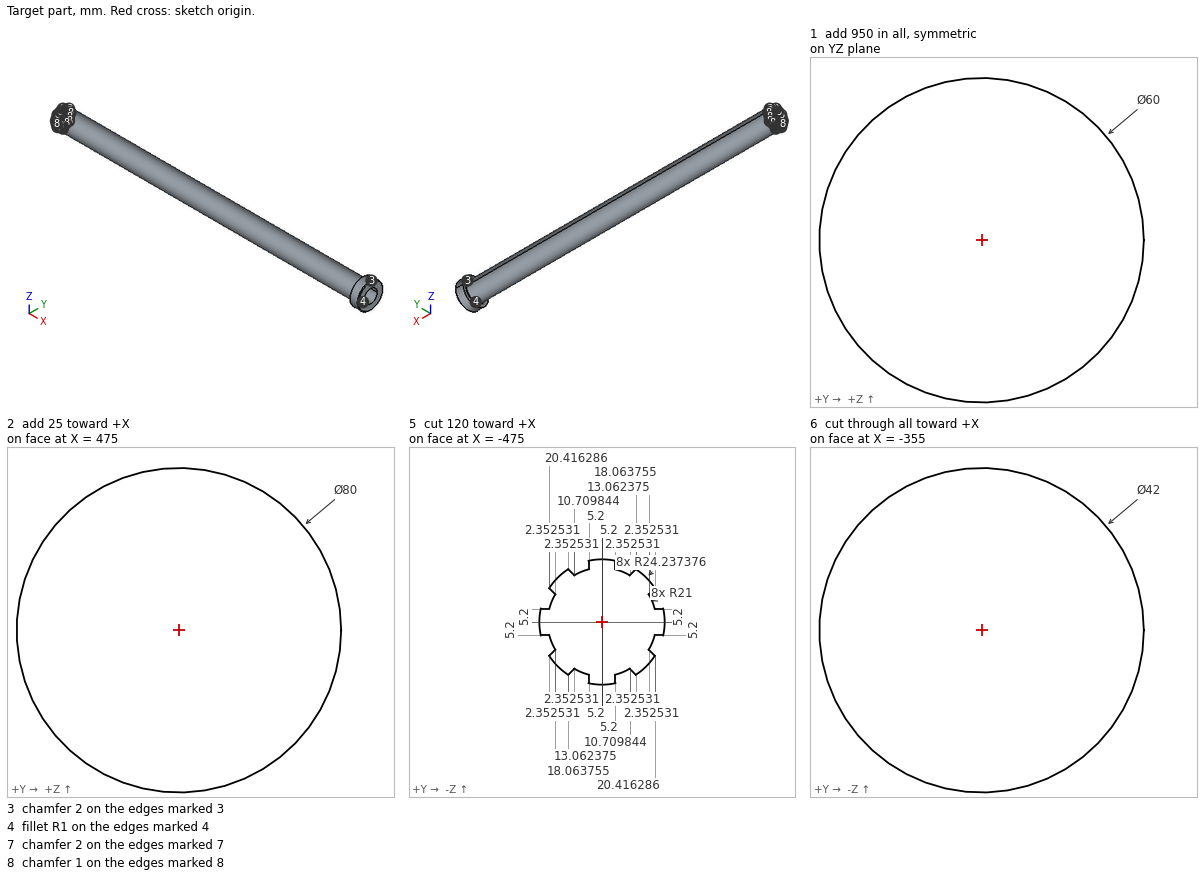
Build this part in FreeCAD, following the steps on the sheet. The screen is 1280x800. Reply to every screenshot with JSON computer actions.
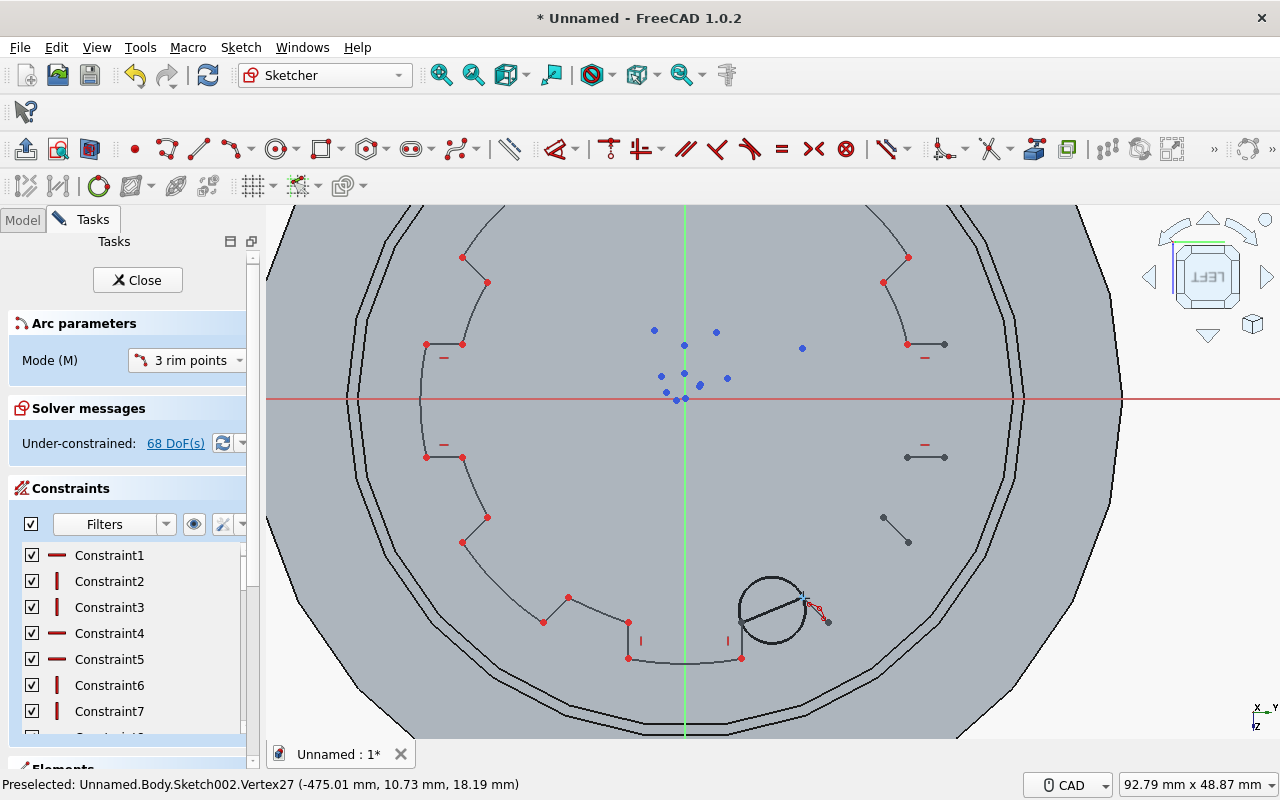
{"action": "scroll", "coordinate": [773, 611], "scroll_direction": "up", "scroll_amount": 10}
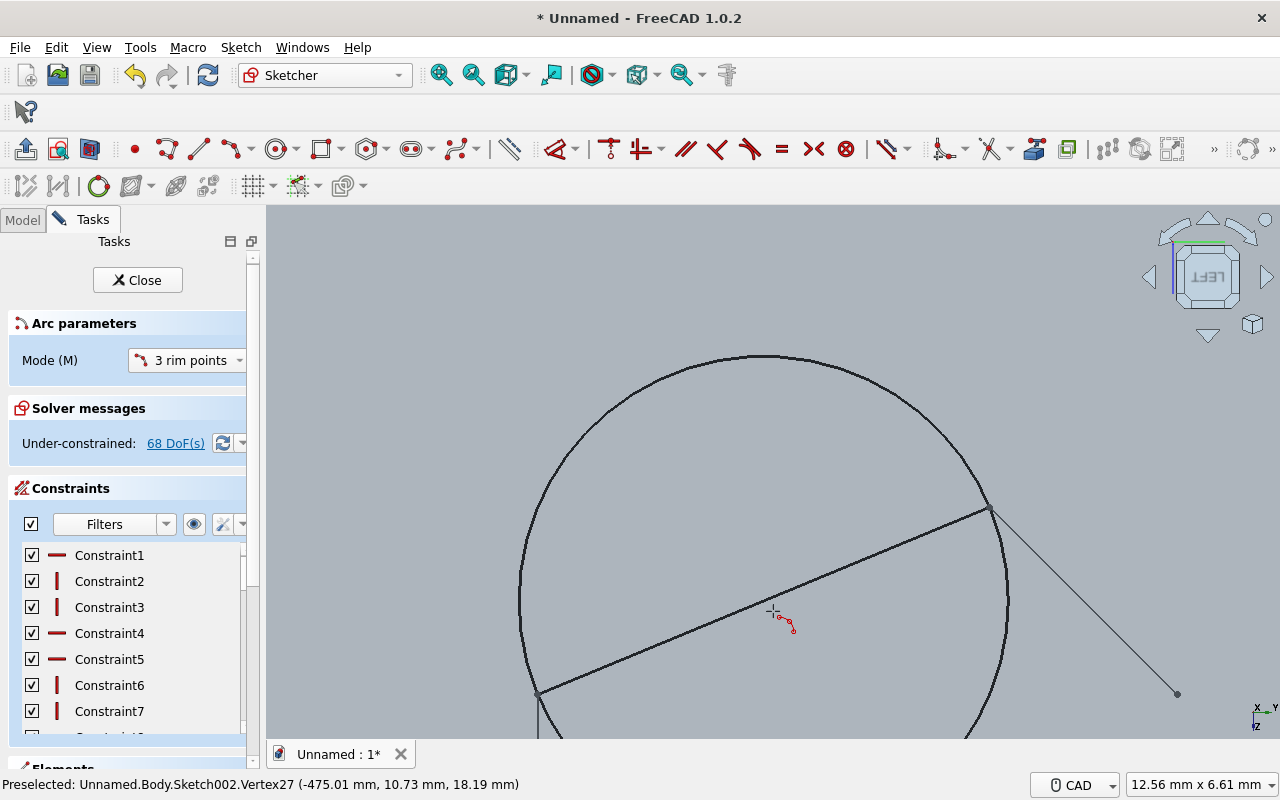
{"action": "left_click", "coordinate": [772, 605]}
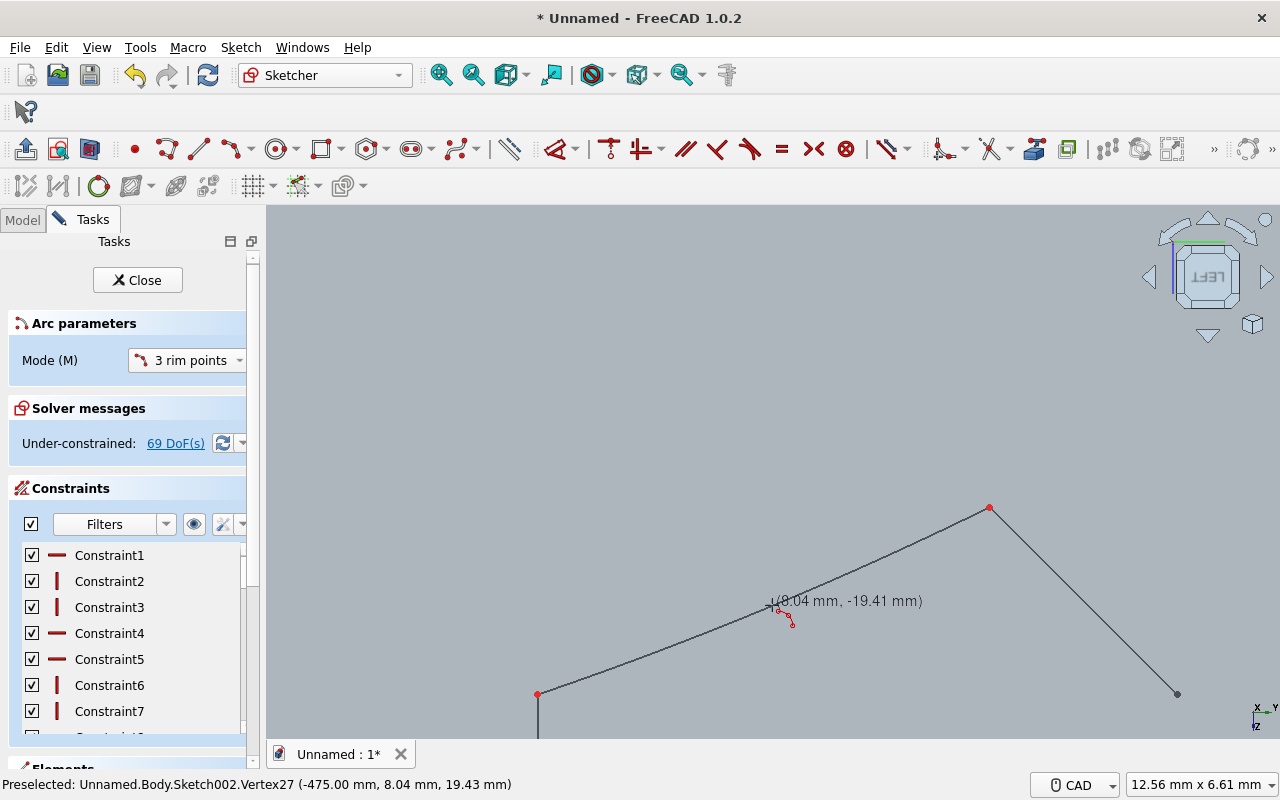
{"action": "scroll", "coordinate": [763, 615], "scroll_direction": "down", "scroll_amount": 12}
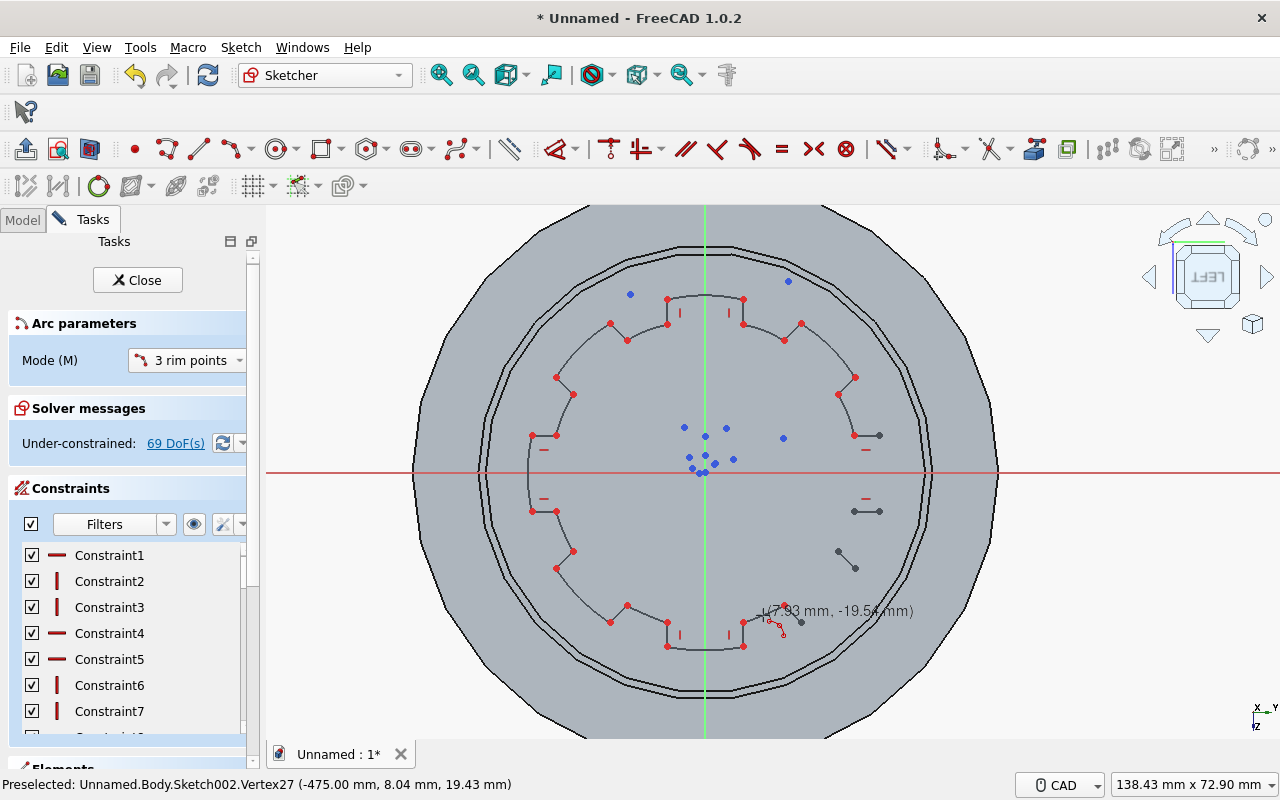
{"action": "scroll", "coordinate": [801, 622], "scroll_direction": "up", "scroll_amount": 2}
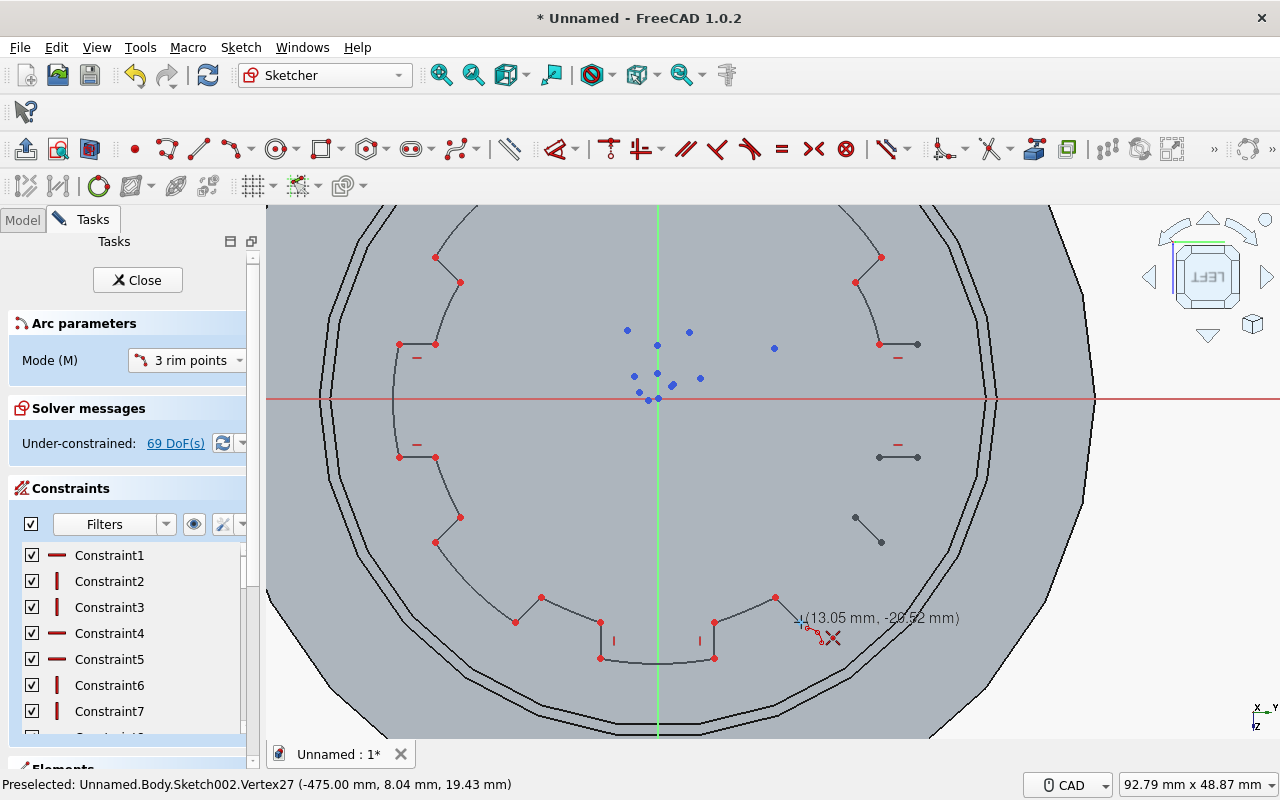
{"action": "left_click", "coordinate": [801, 623]}
{"action": "left_click", "coordinate": [881, 542]}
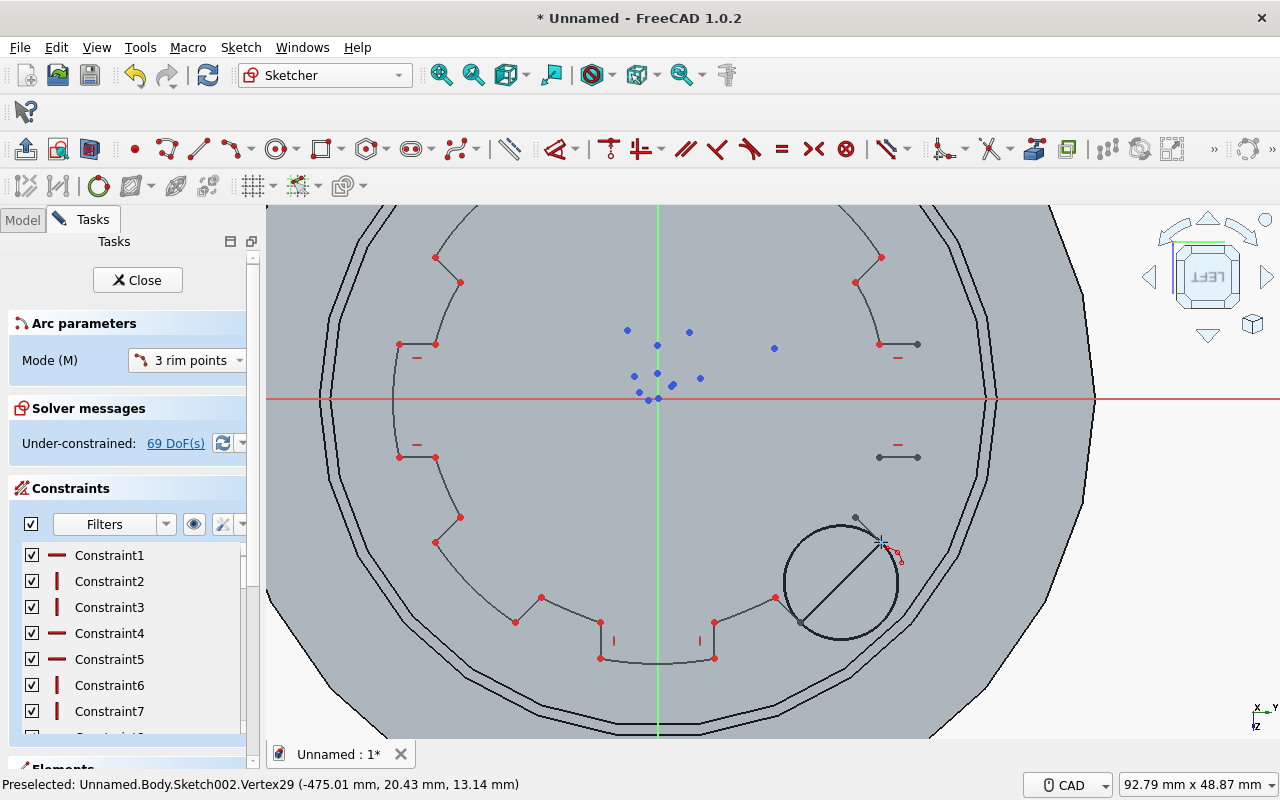
{"action": "scroll", "coordinate": [845, 586], "scroll_direction": "up", "scroll_amount": 5}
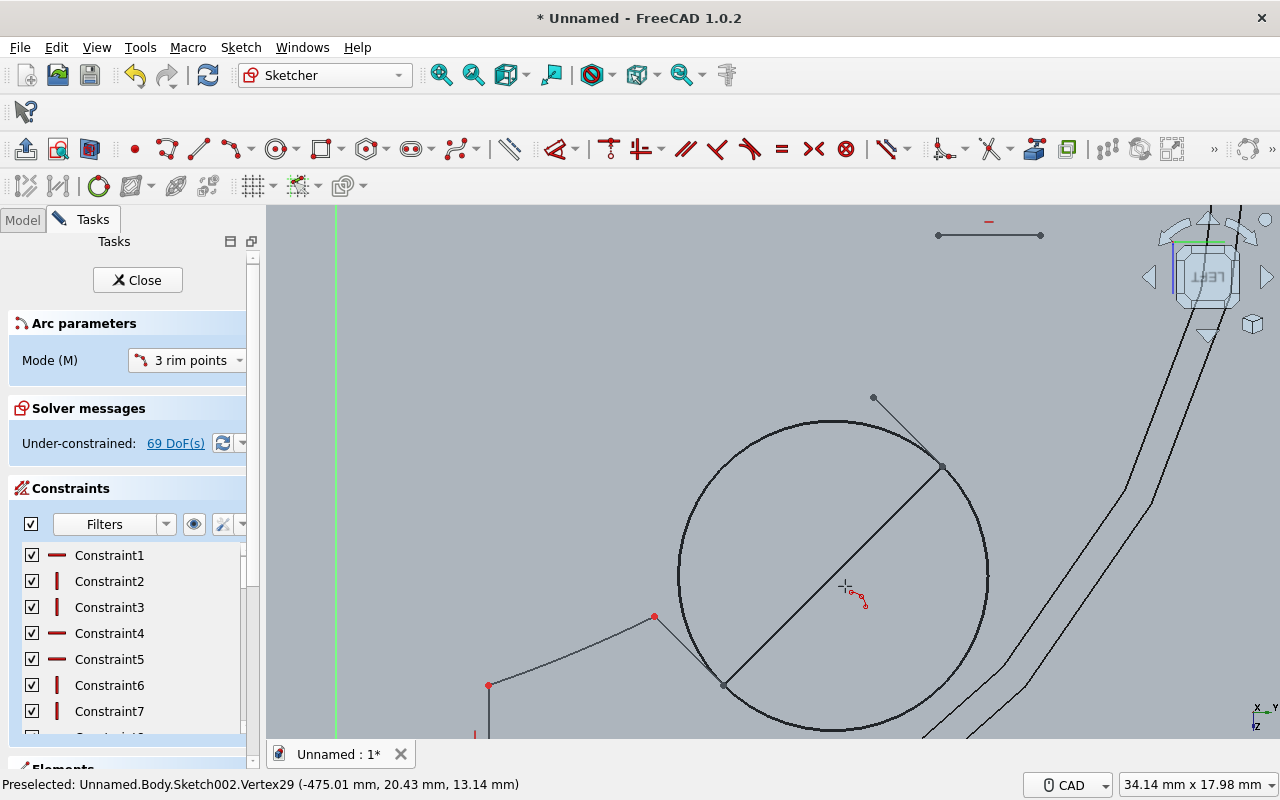
{"action": "left_click", "coordinate": [845, 585]}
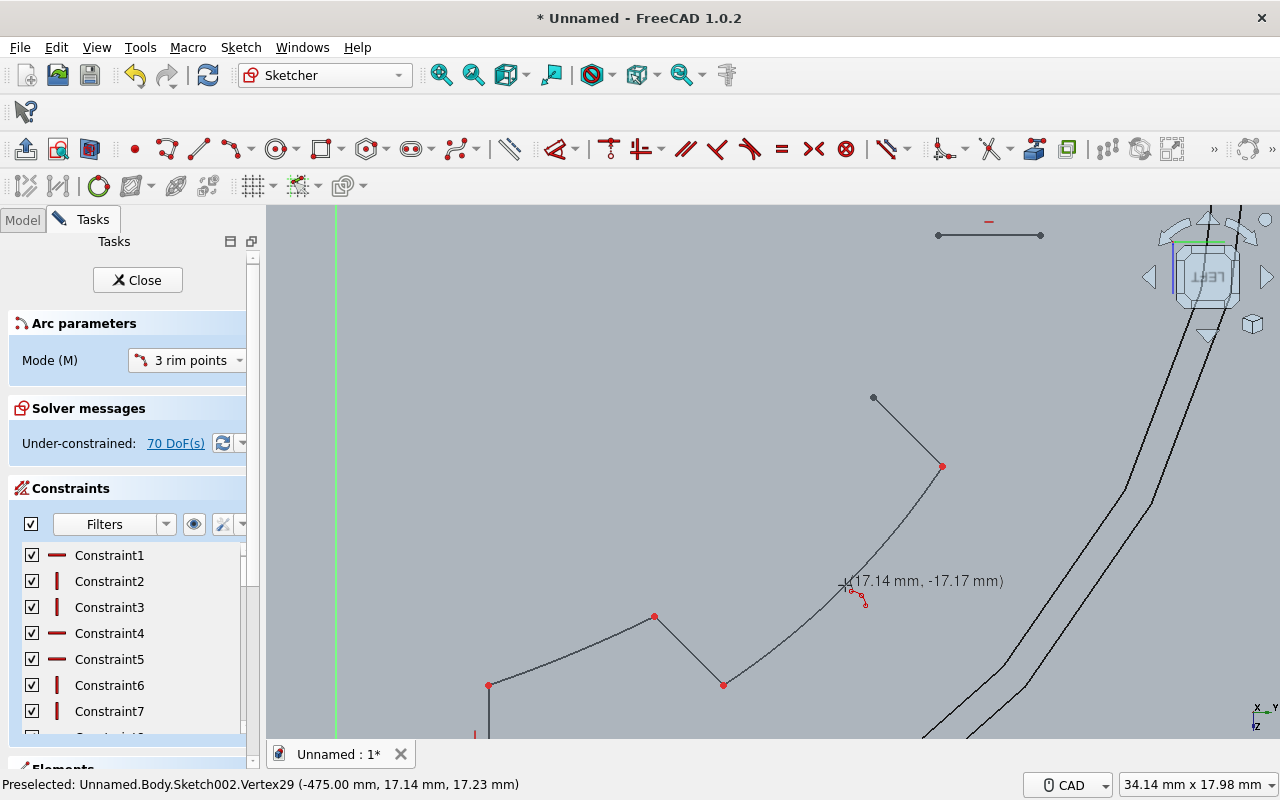
{"action": "scroll", "coordinate": [825, 602], "scroll_direction": "down", "scroll_amount": 7}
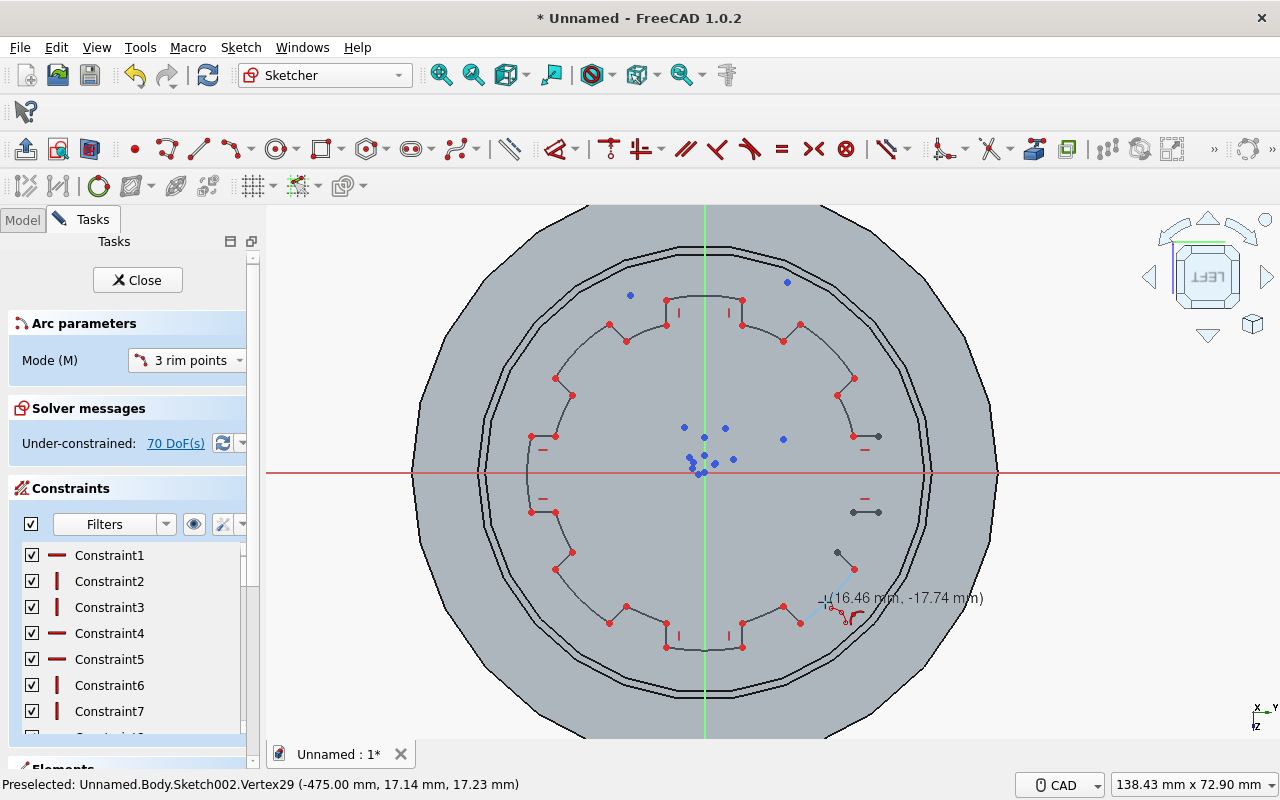
{"action": "scroll", "coordinate": [837, 551], "scroll_direction": "up", "scroll_amount": 2}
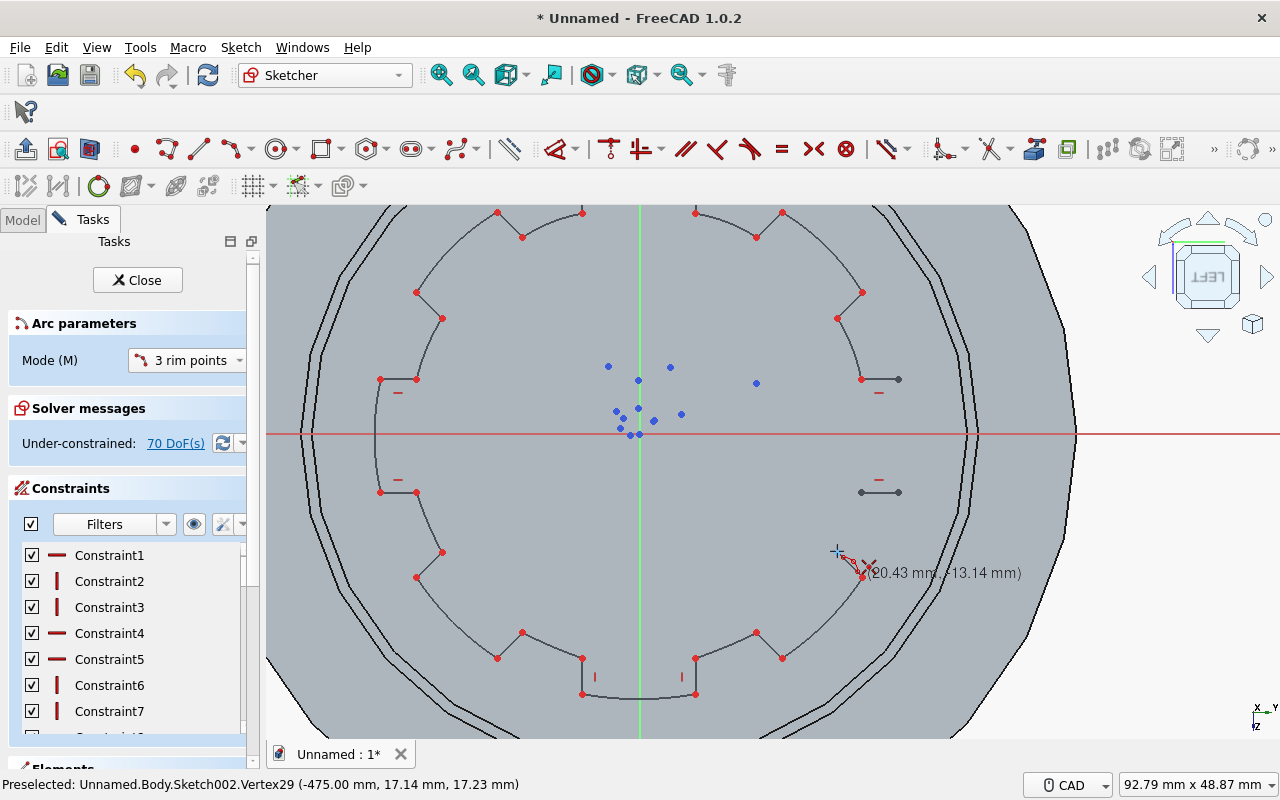
{"action": "left_click", "coordinate": [837, 552]}
{"action": "left_click", "coordinate": [861, 493]}